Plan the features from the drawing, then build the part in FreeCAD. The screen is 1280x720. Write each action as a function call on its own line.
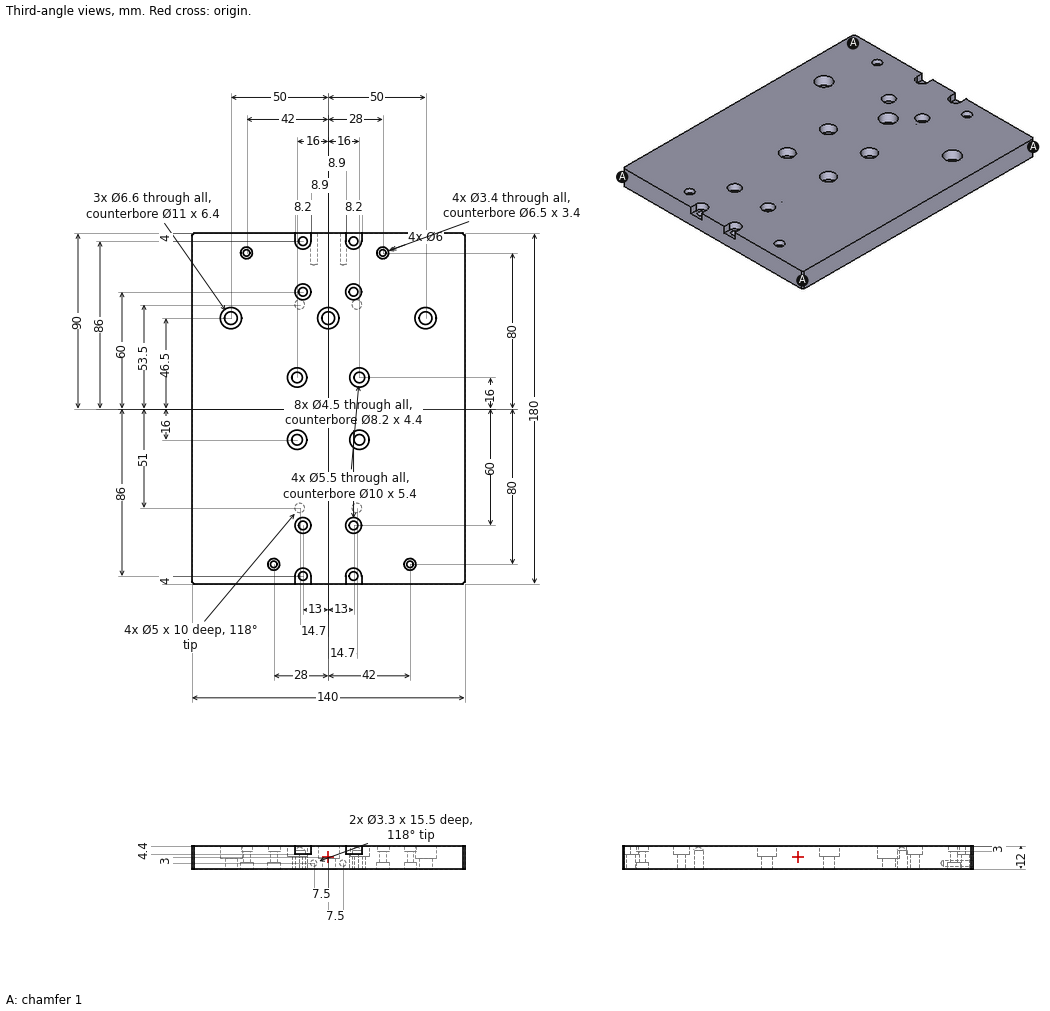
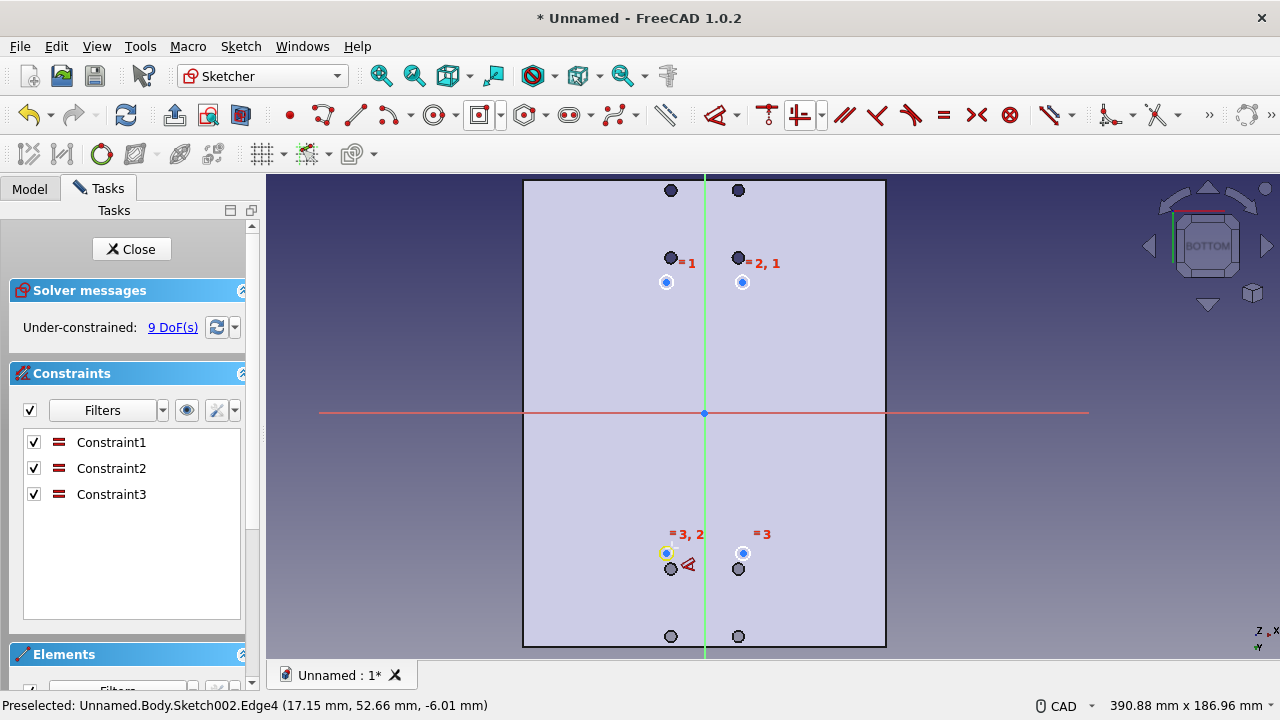
scroll(671, 277, up, 6)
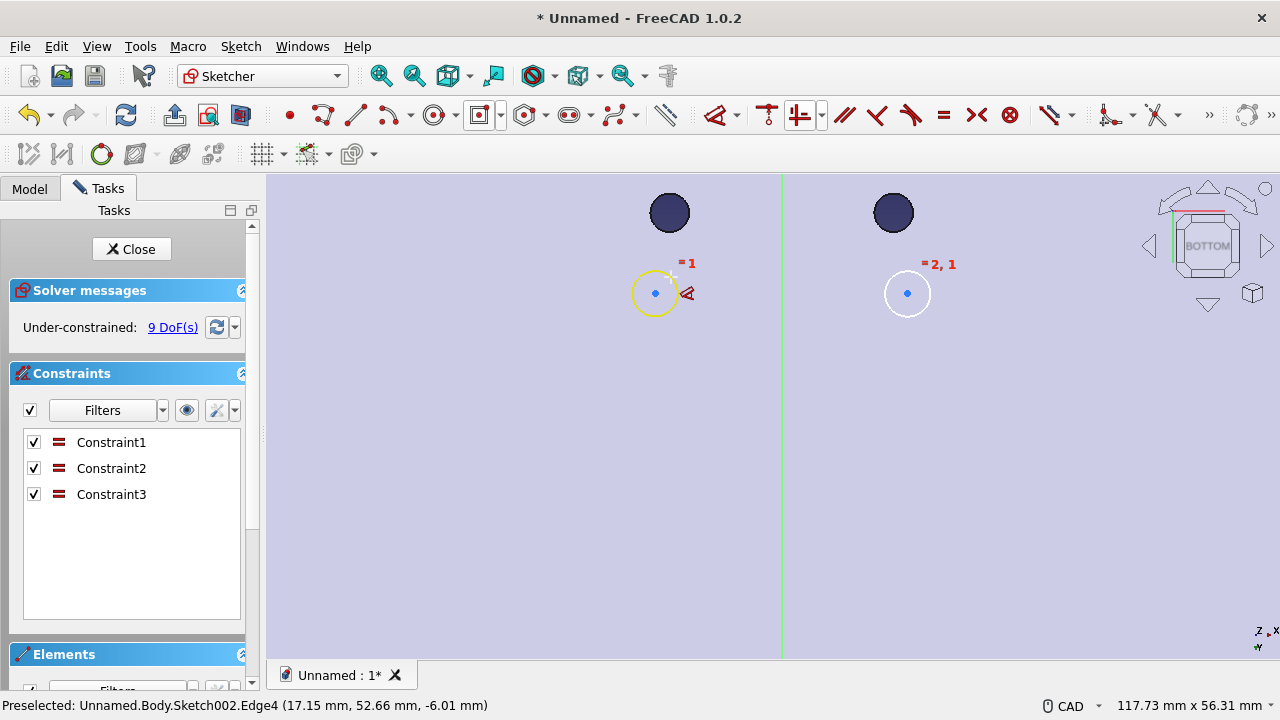
click(671, 278)
click(694, 255)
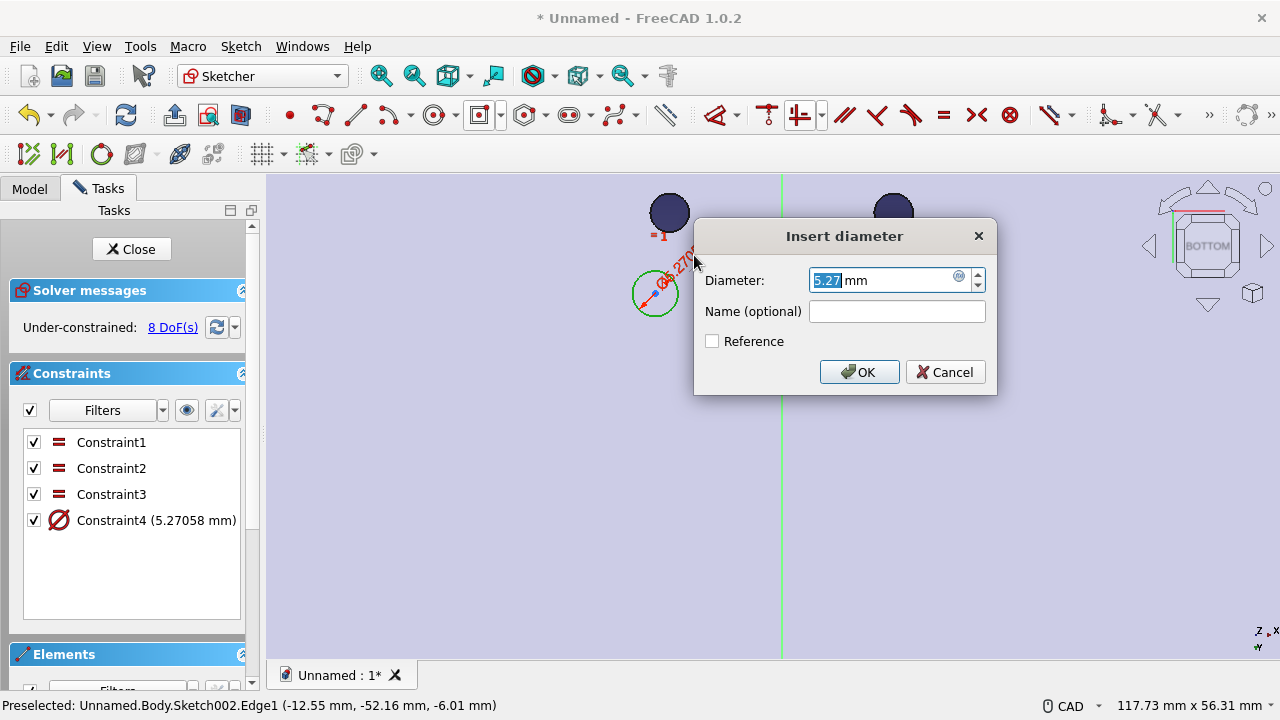
text(5)
key(Return)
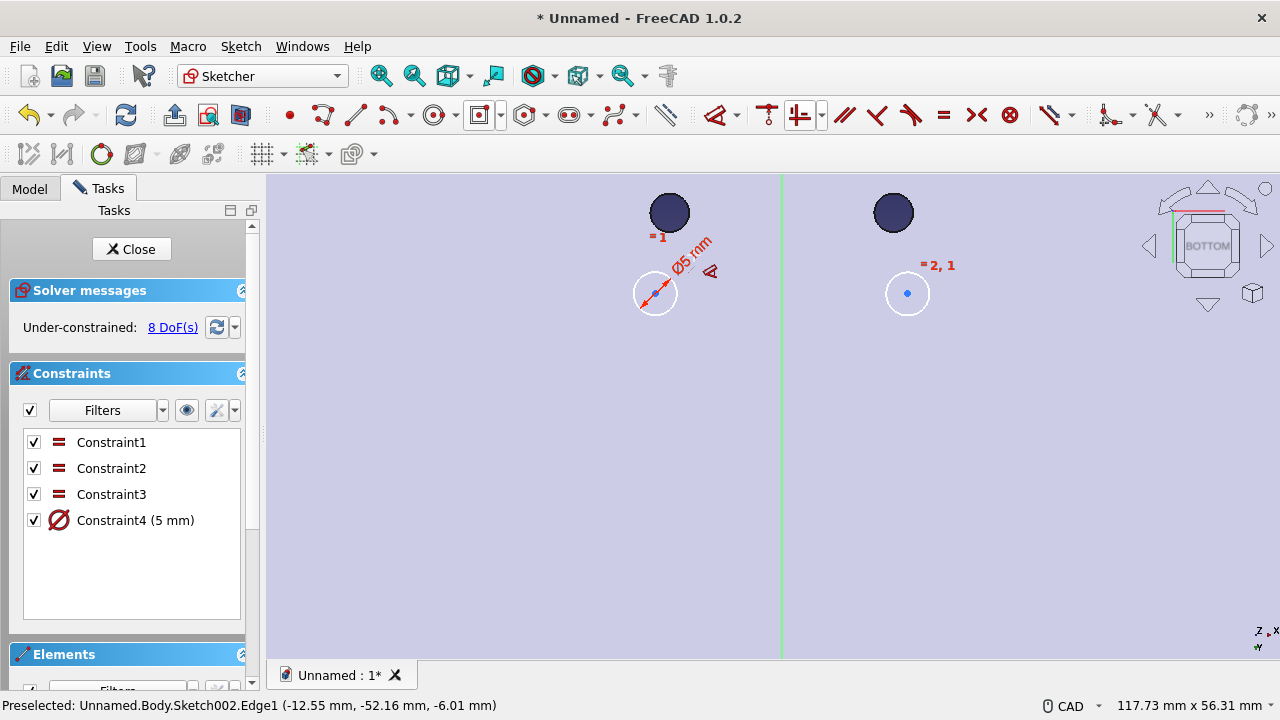
scroll(671, 277, down, 6)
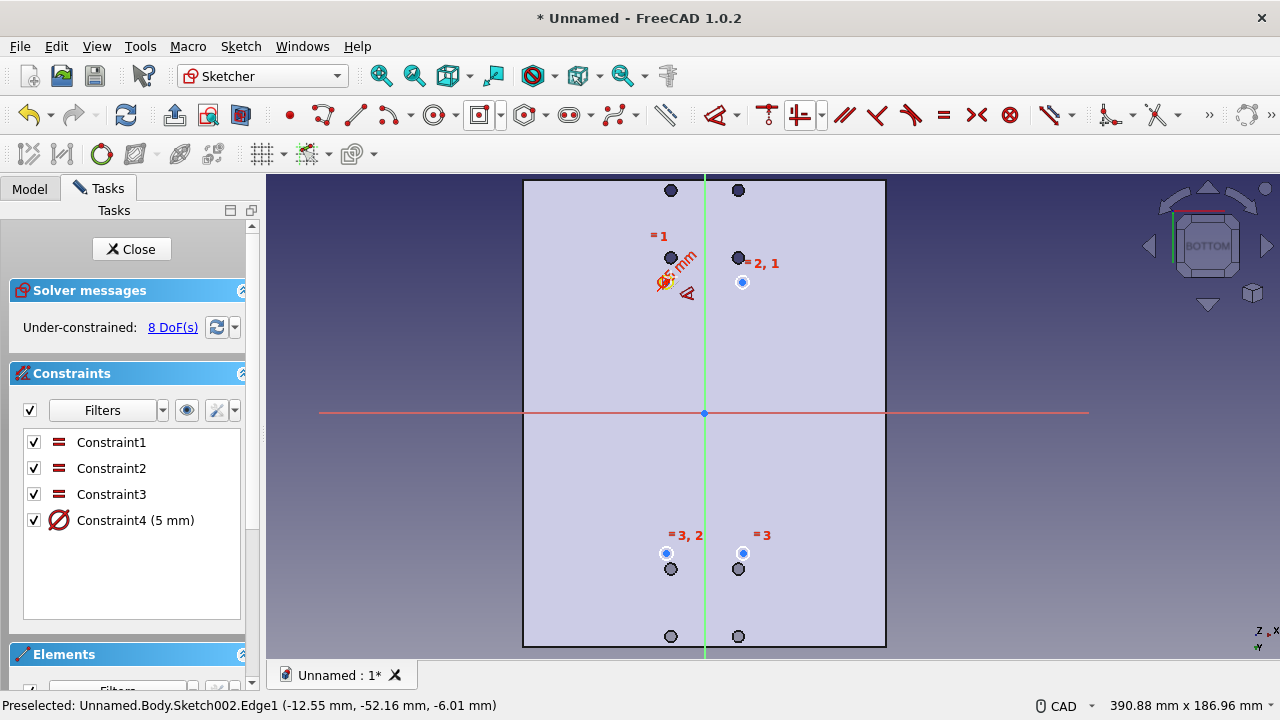
click(667, 282)
click(633, 348)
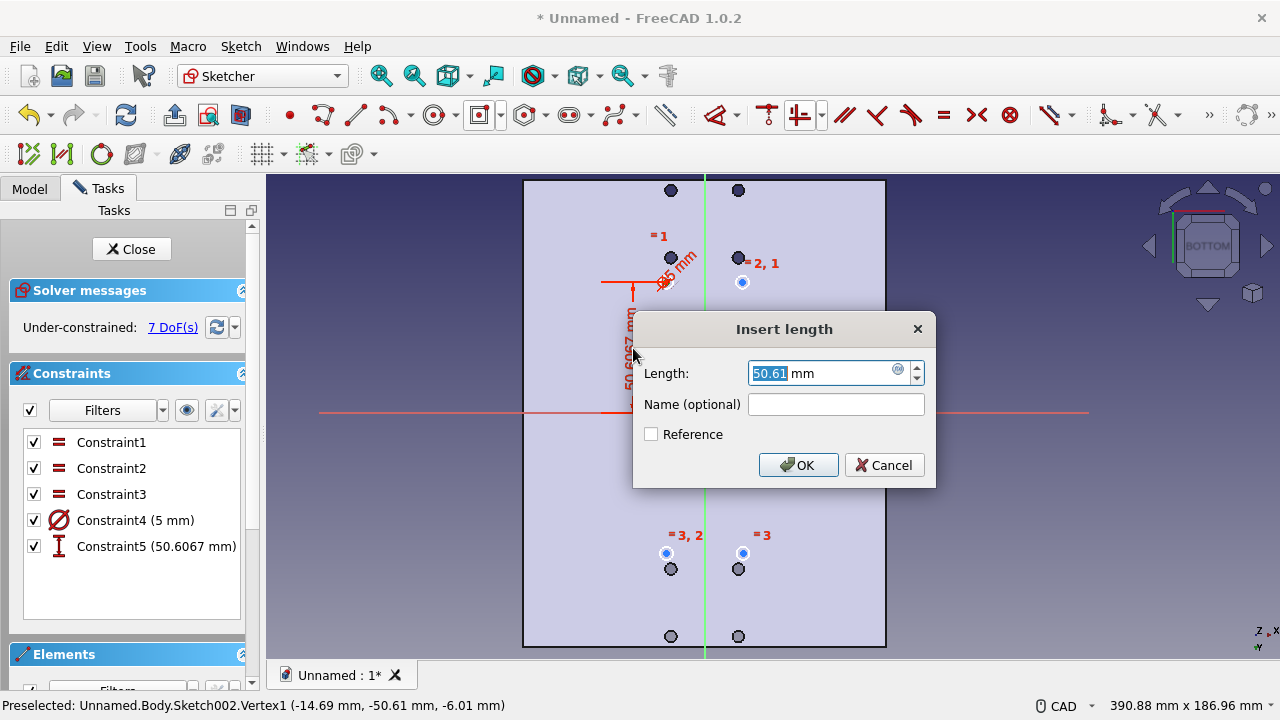
text(51)
key(Return)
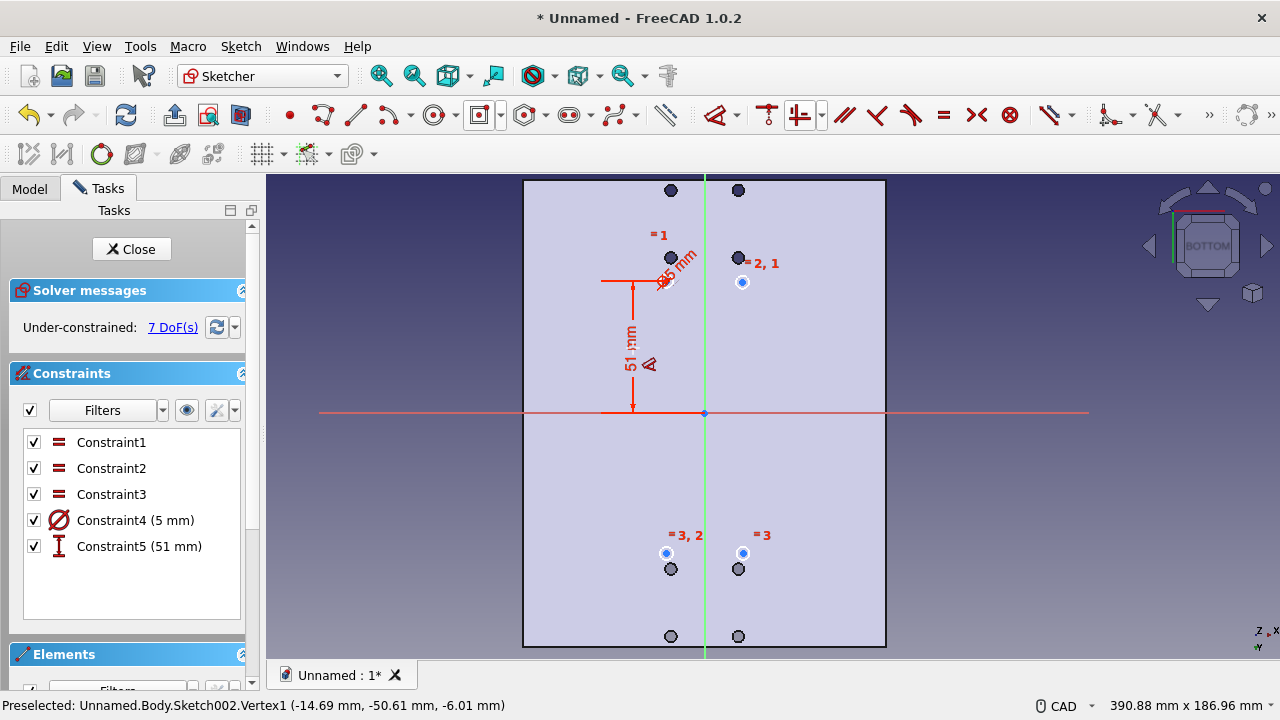
click(743, 282)
click(777, 348)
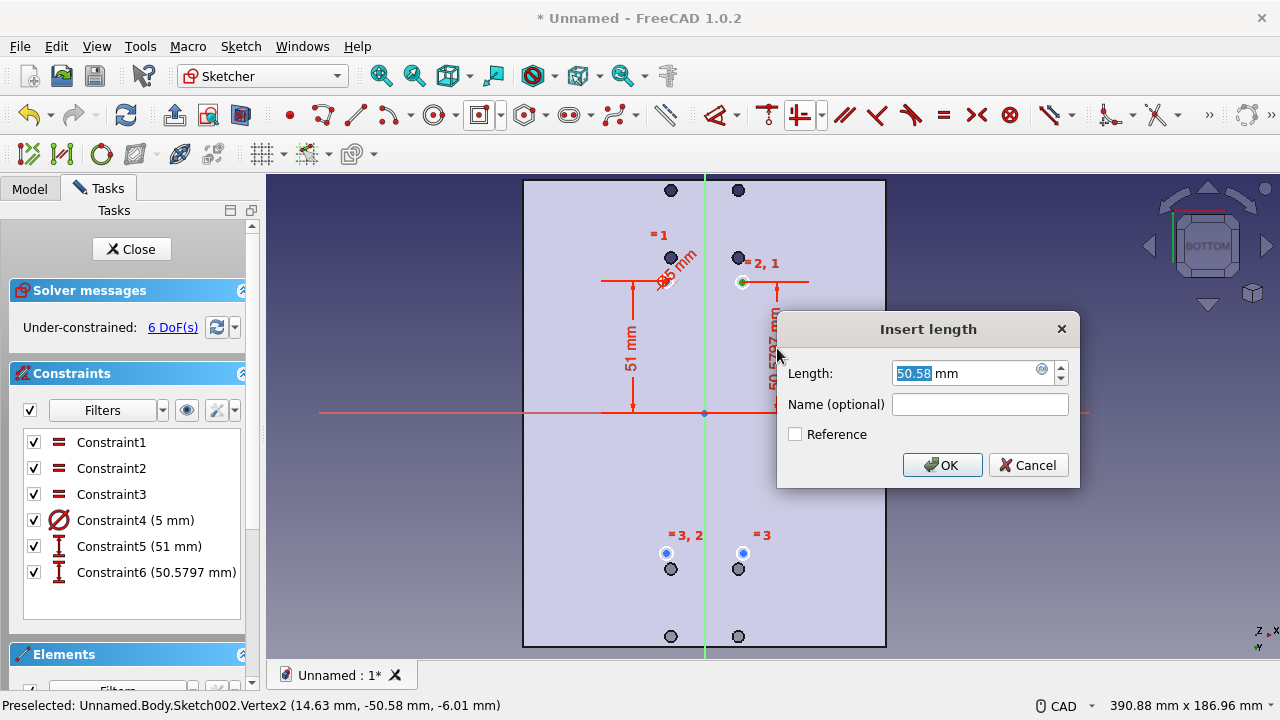
text(51)
key(Return)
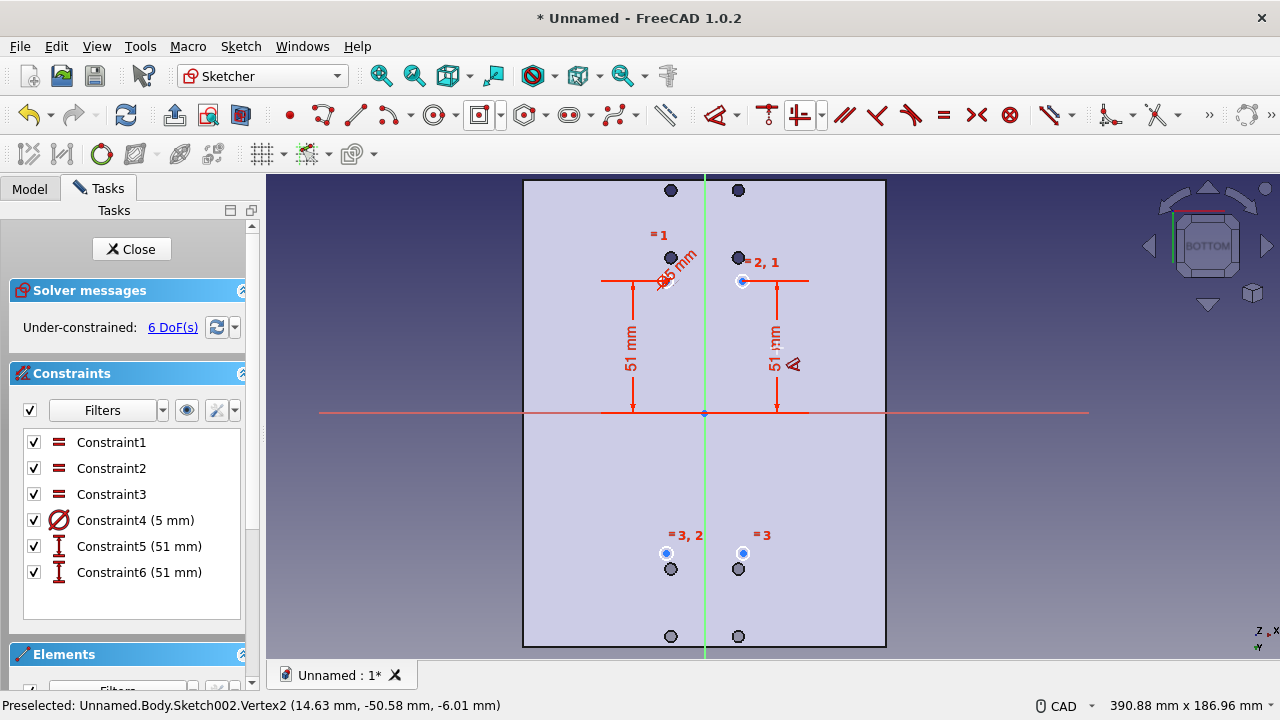
click(667, 281)
click(686, 247)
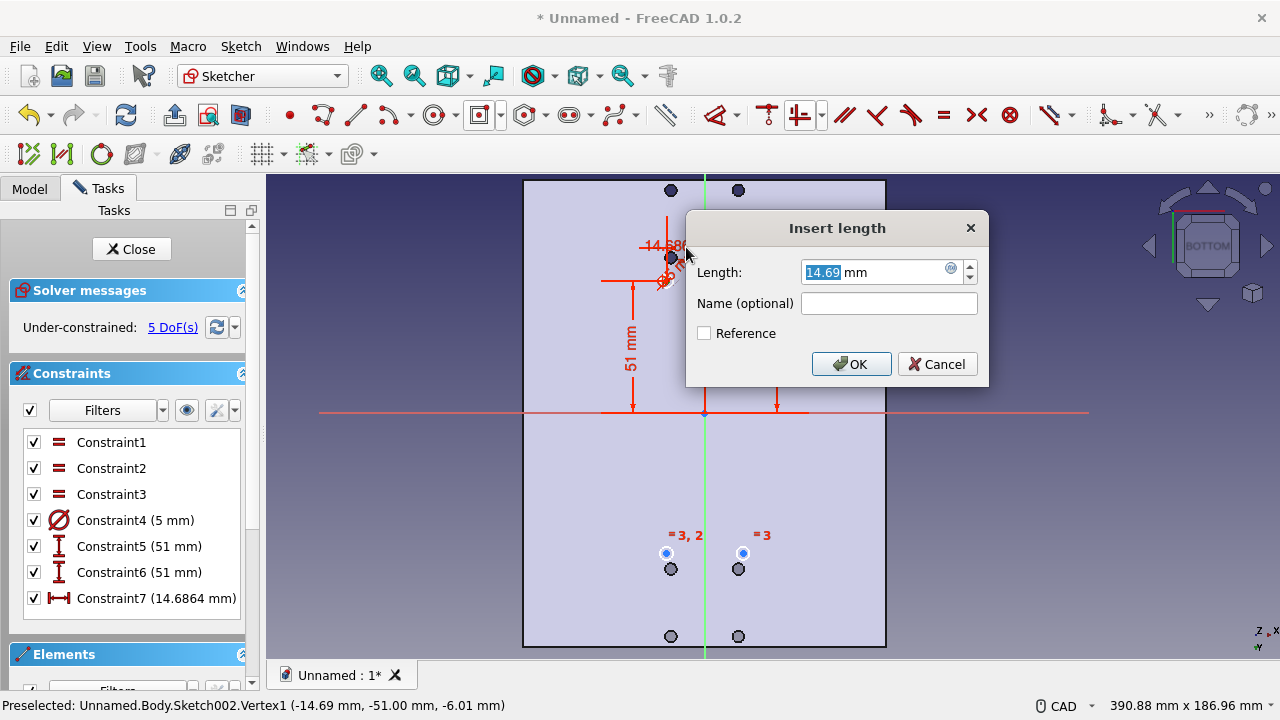
text(14.7)
key(Return)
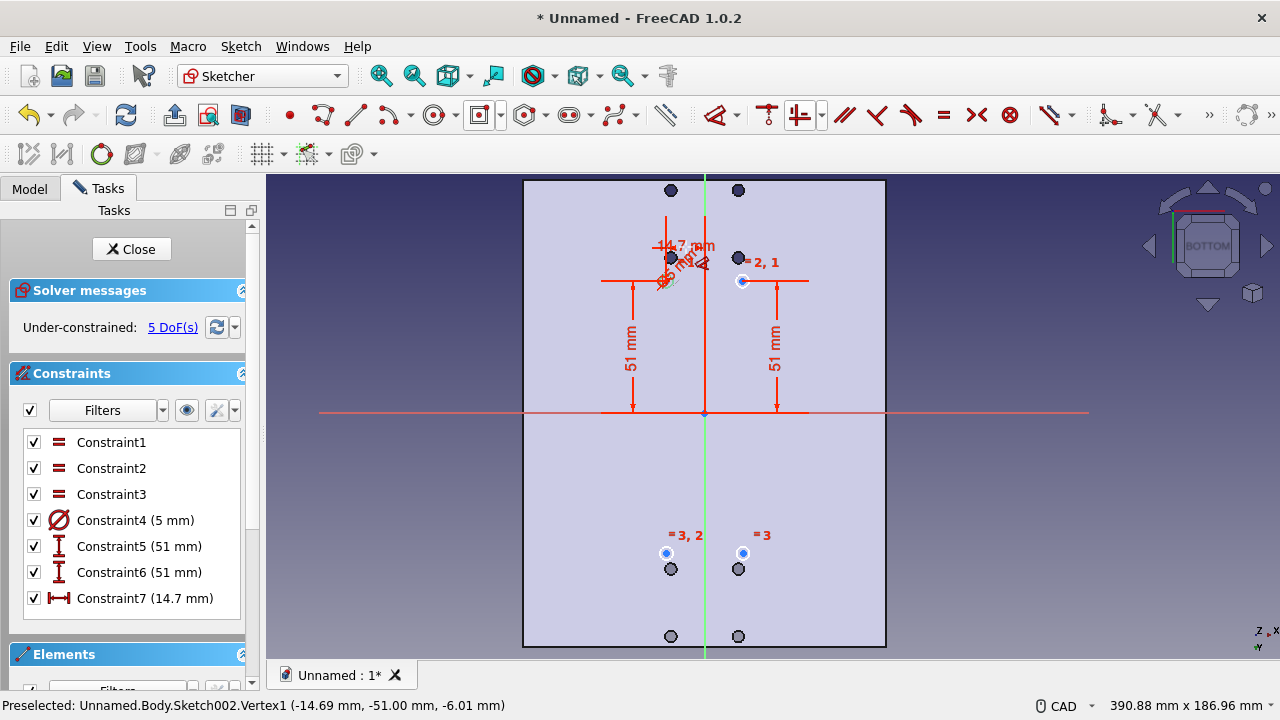
click(743, 281)
click(724, 447)